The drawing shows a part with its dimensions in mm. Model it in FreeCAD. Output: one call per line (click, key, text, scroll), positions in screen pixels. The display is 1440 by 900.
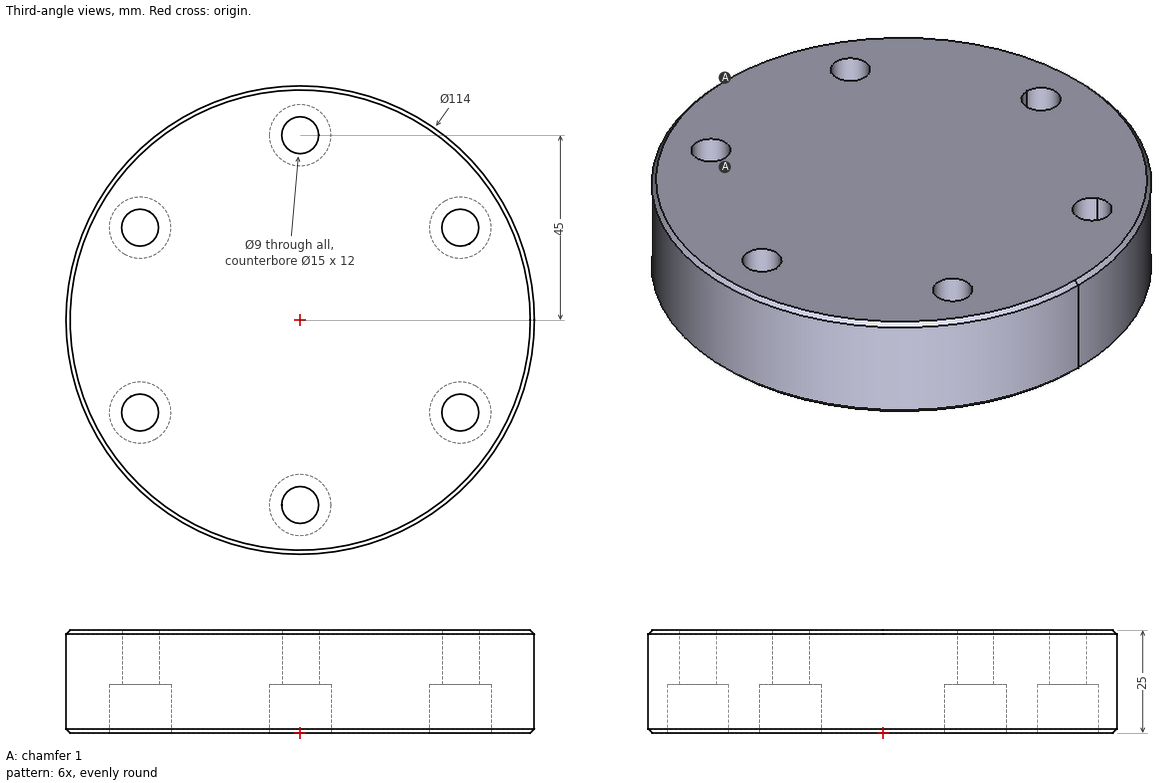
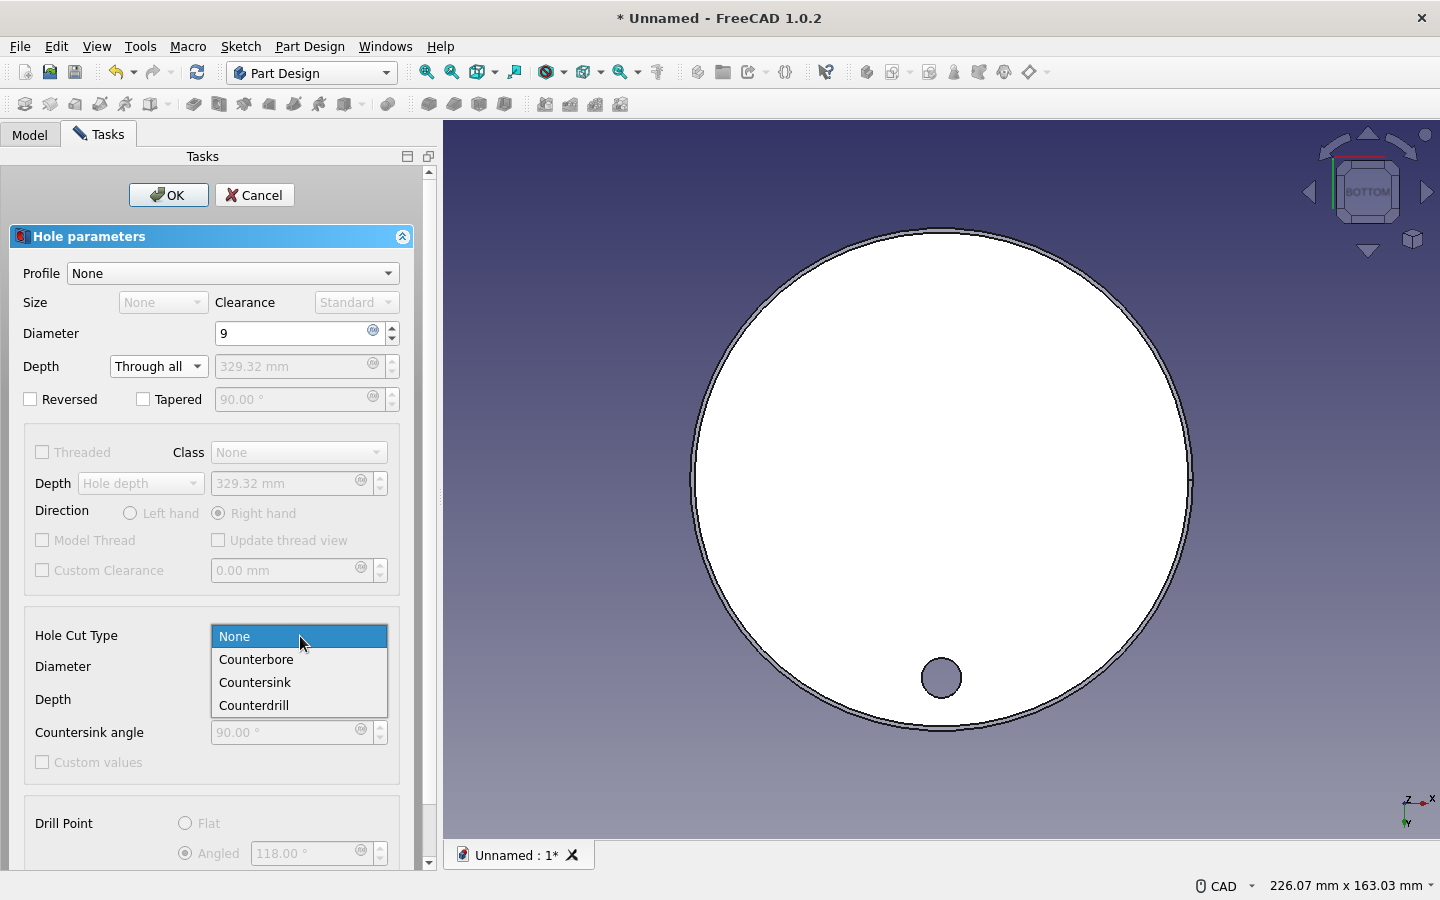
click(298, 660)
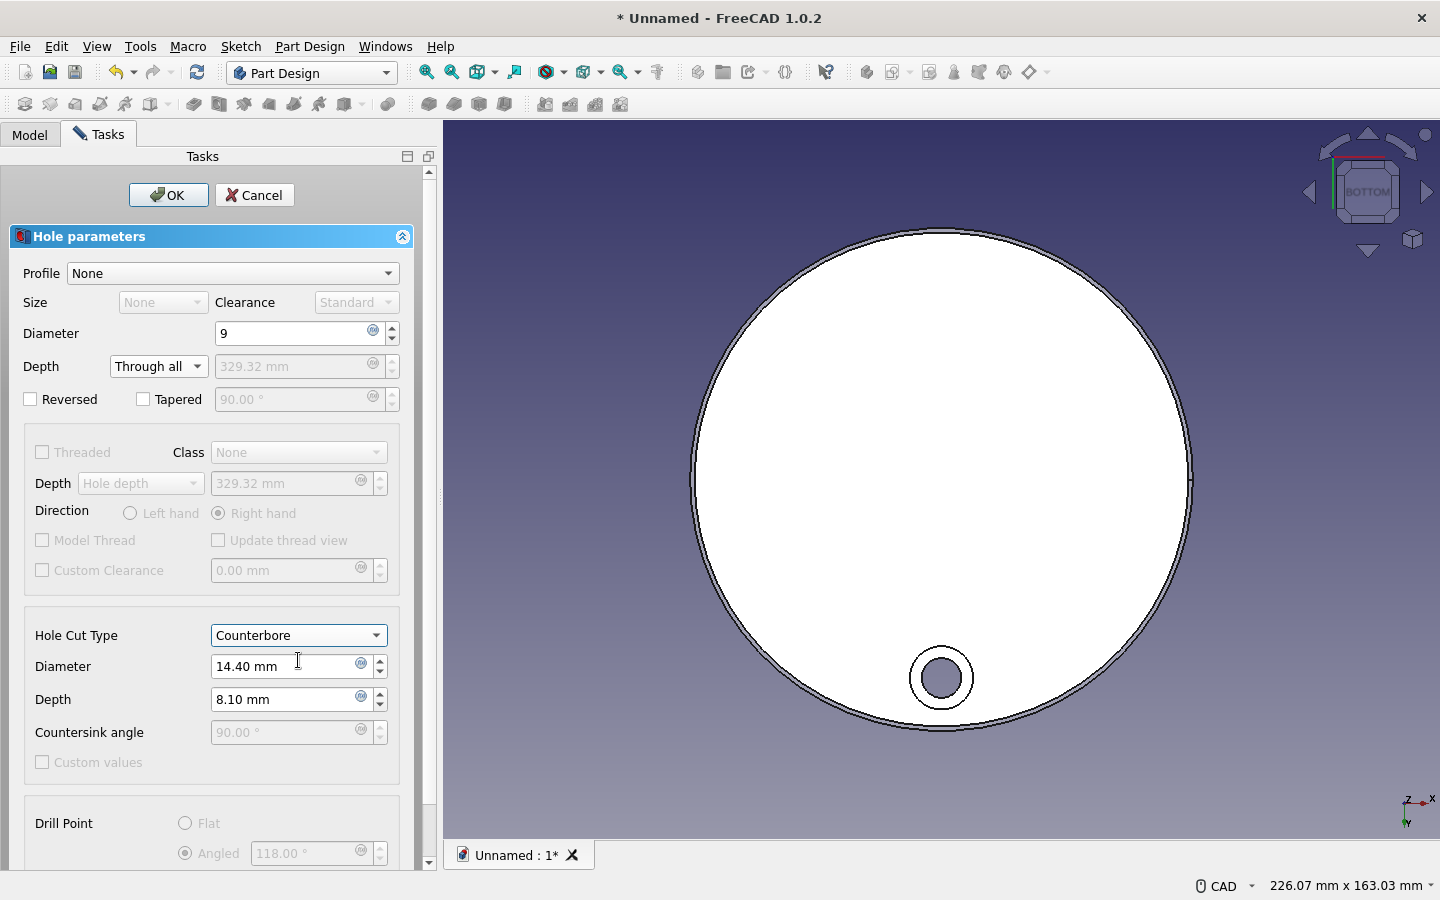
triple_click(292, 666)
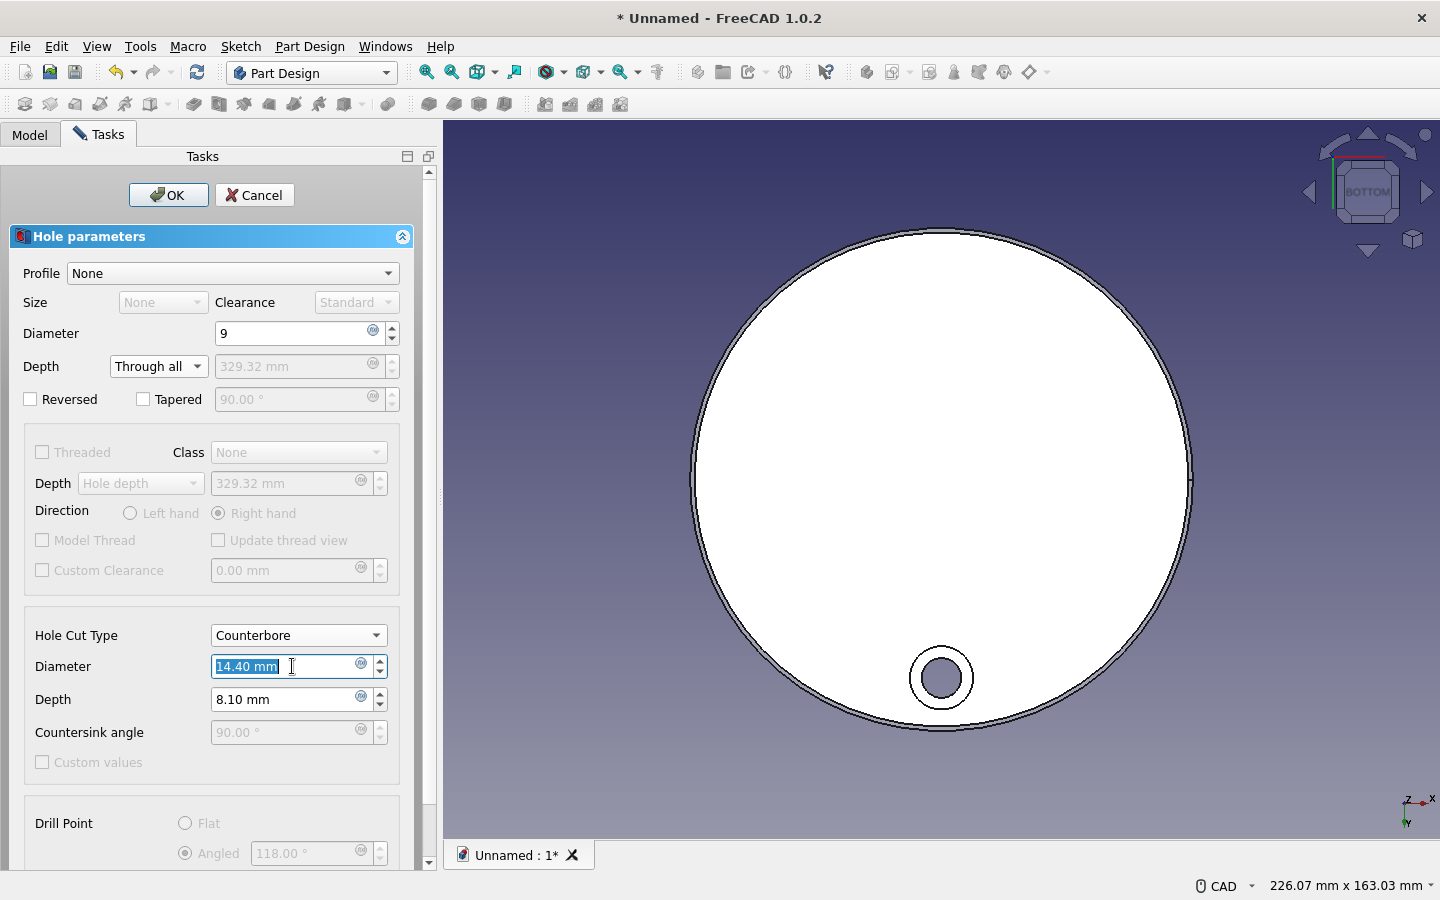
text(15)
key(Tab)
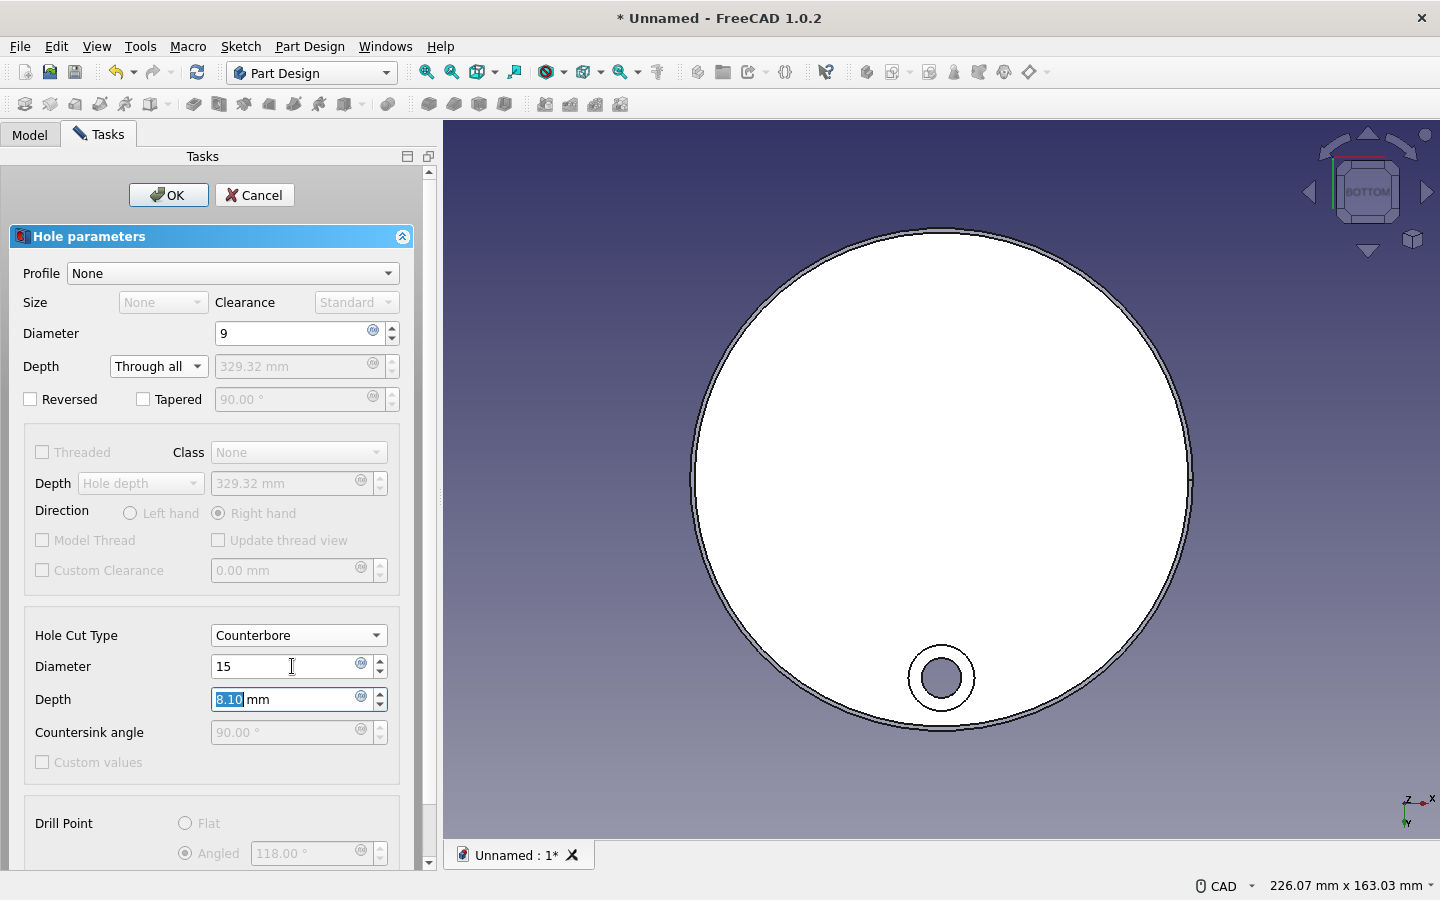
text(12)
key(Tab)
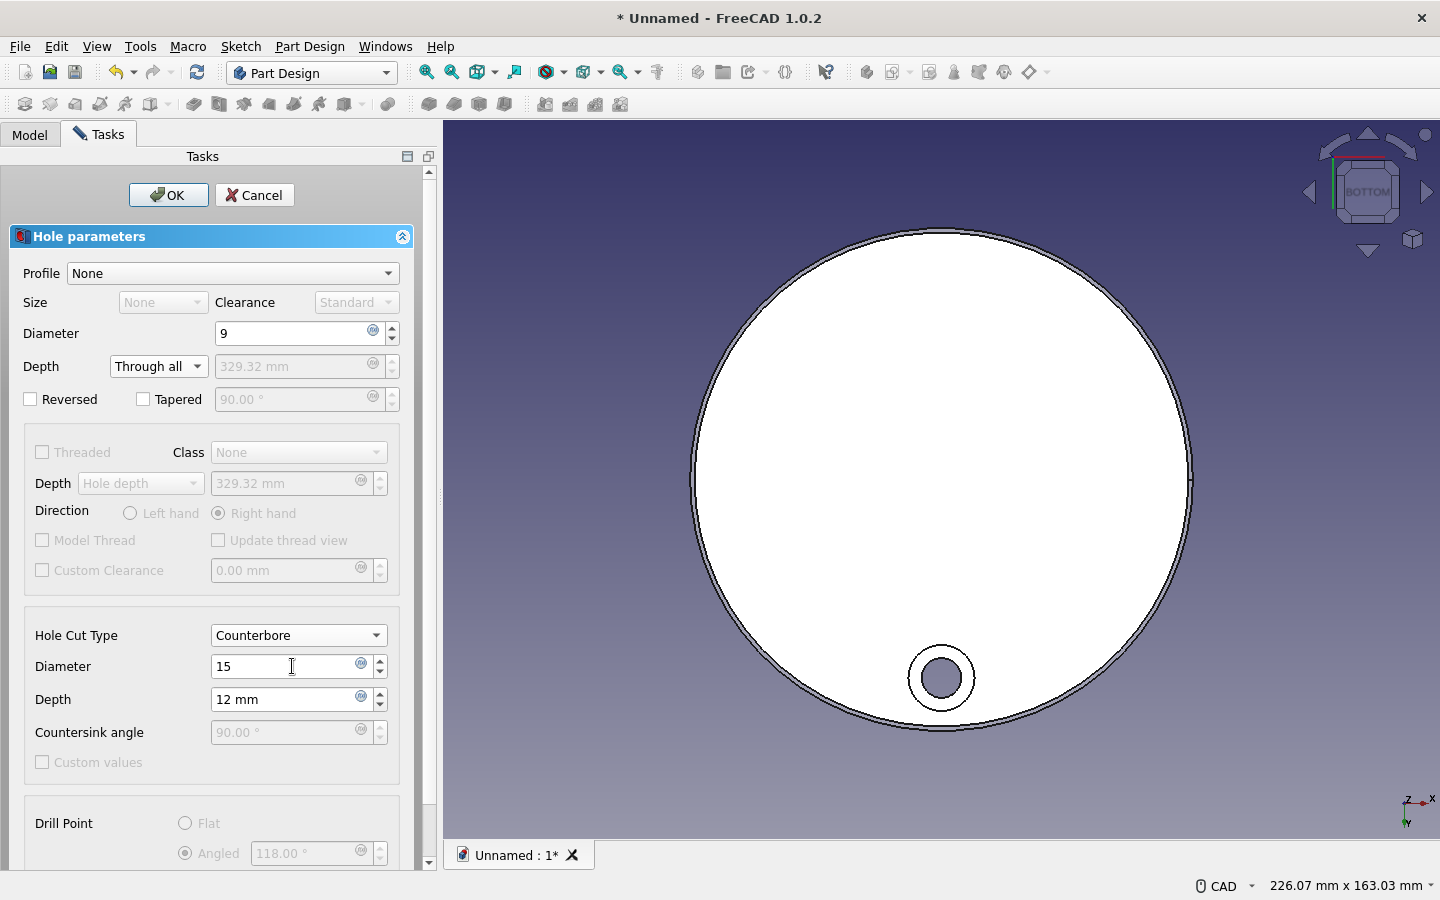
click(169, 195)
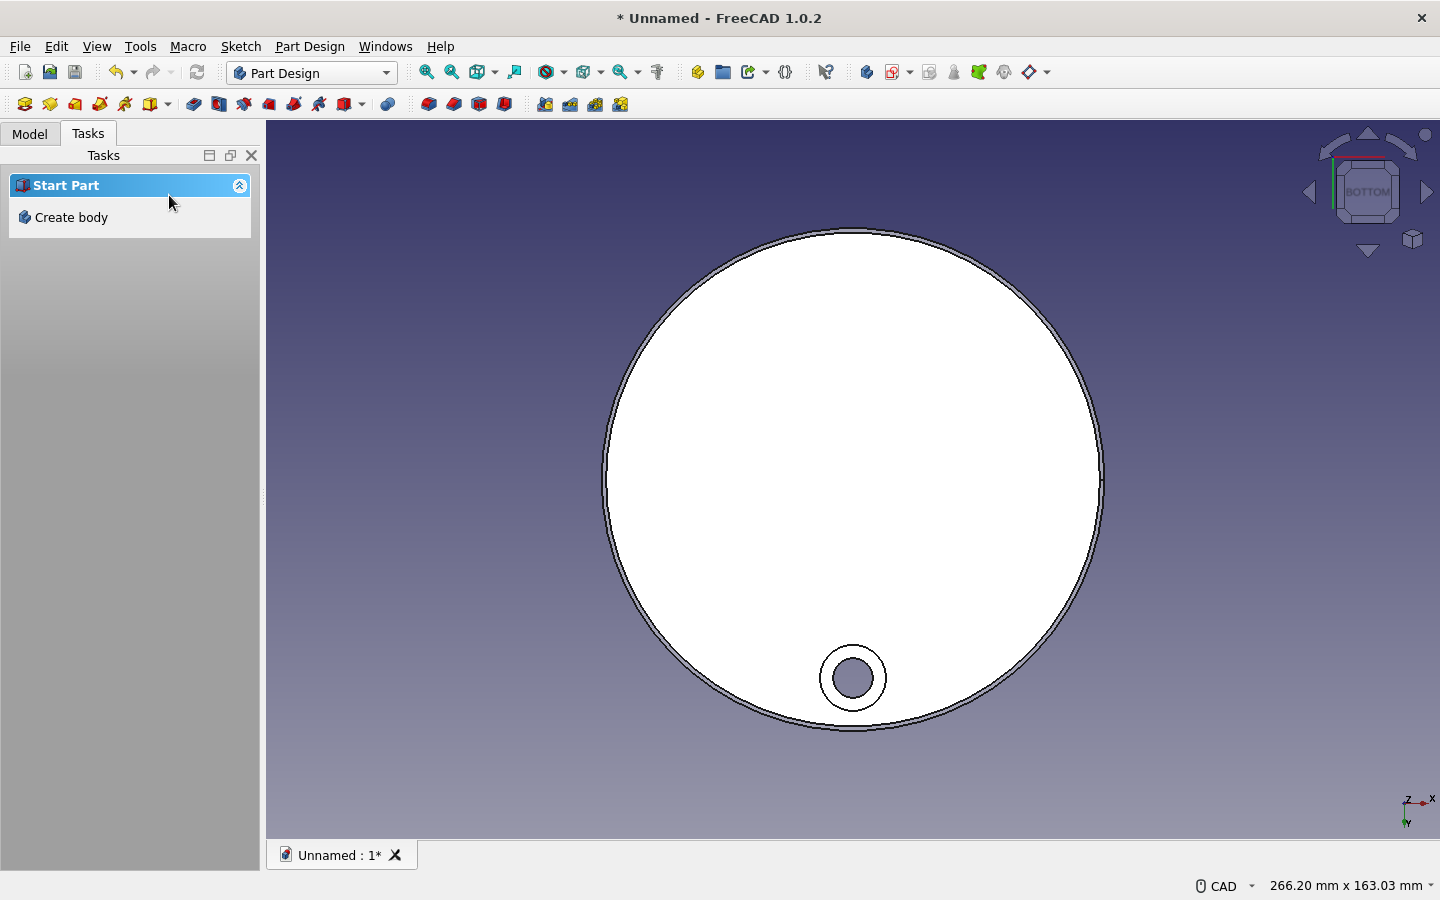
click(30, 134)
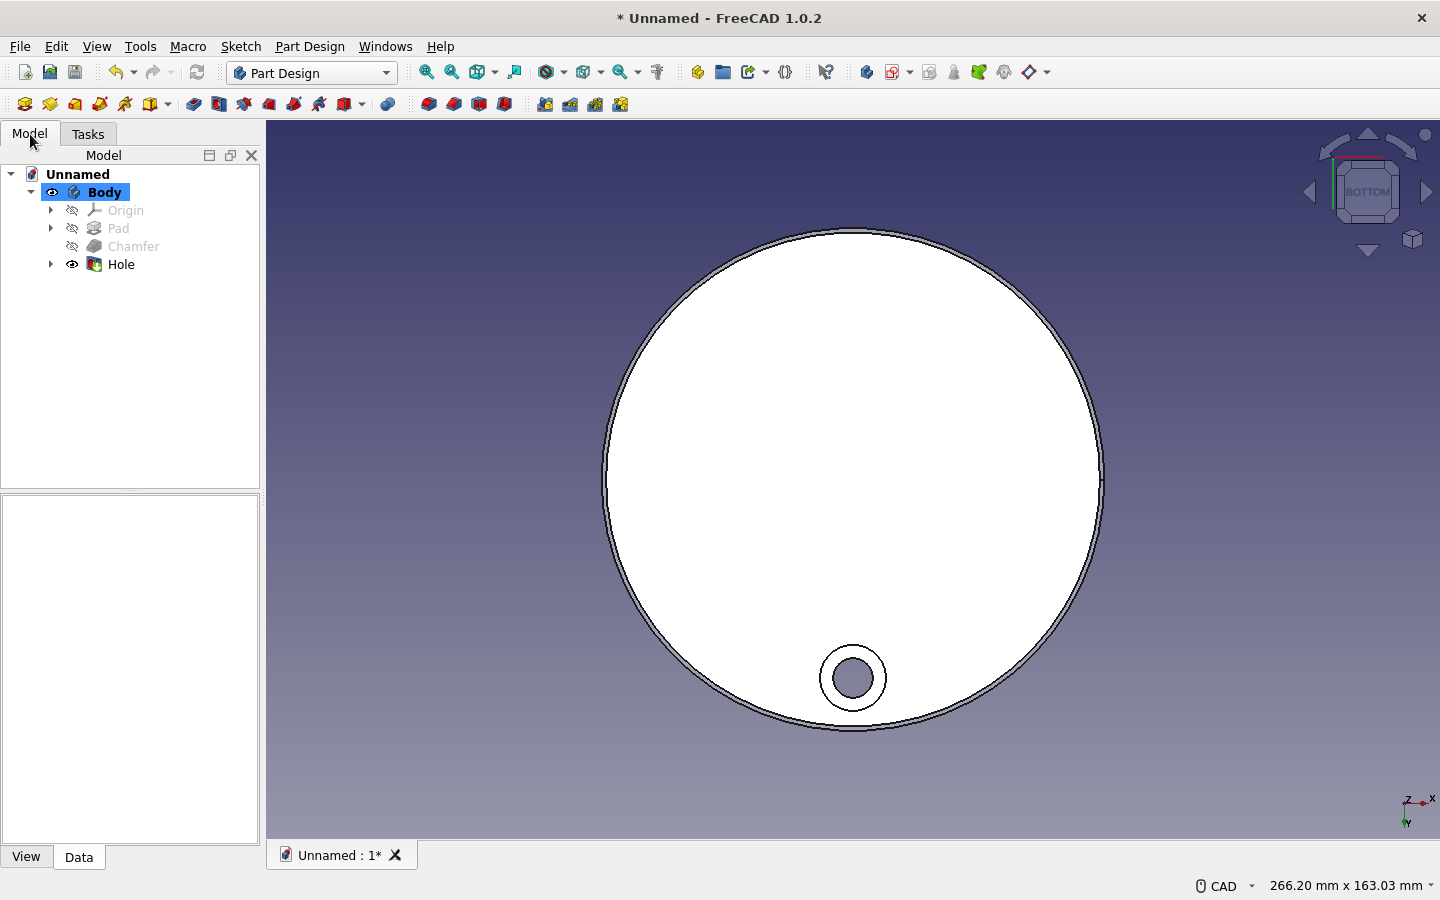
click(117, 264)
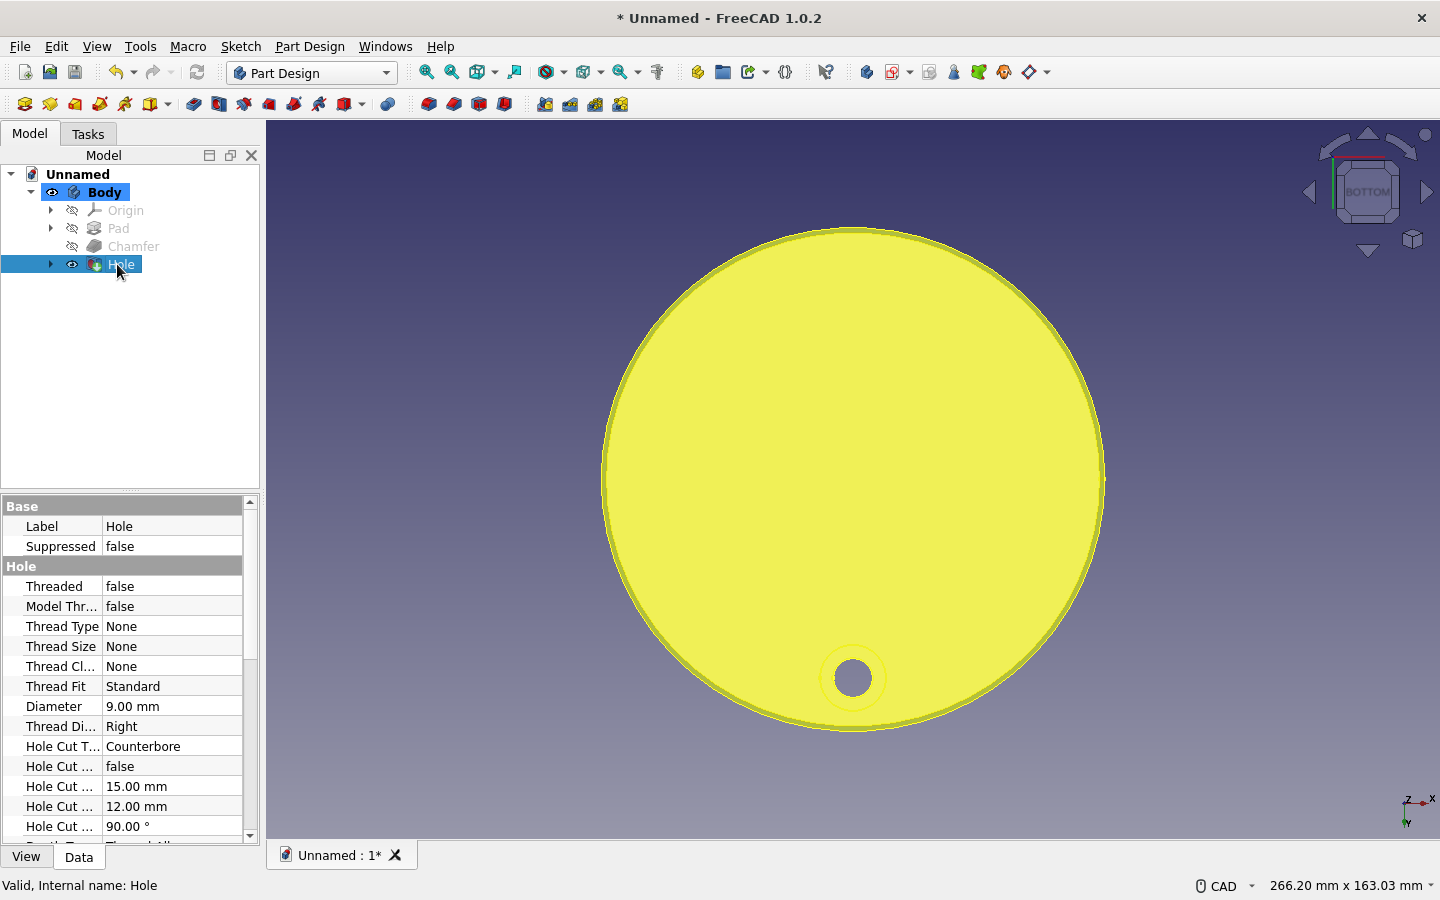
click(595, 104)